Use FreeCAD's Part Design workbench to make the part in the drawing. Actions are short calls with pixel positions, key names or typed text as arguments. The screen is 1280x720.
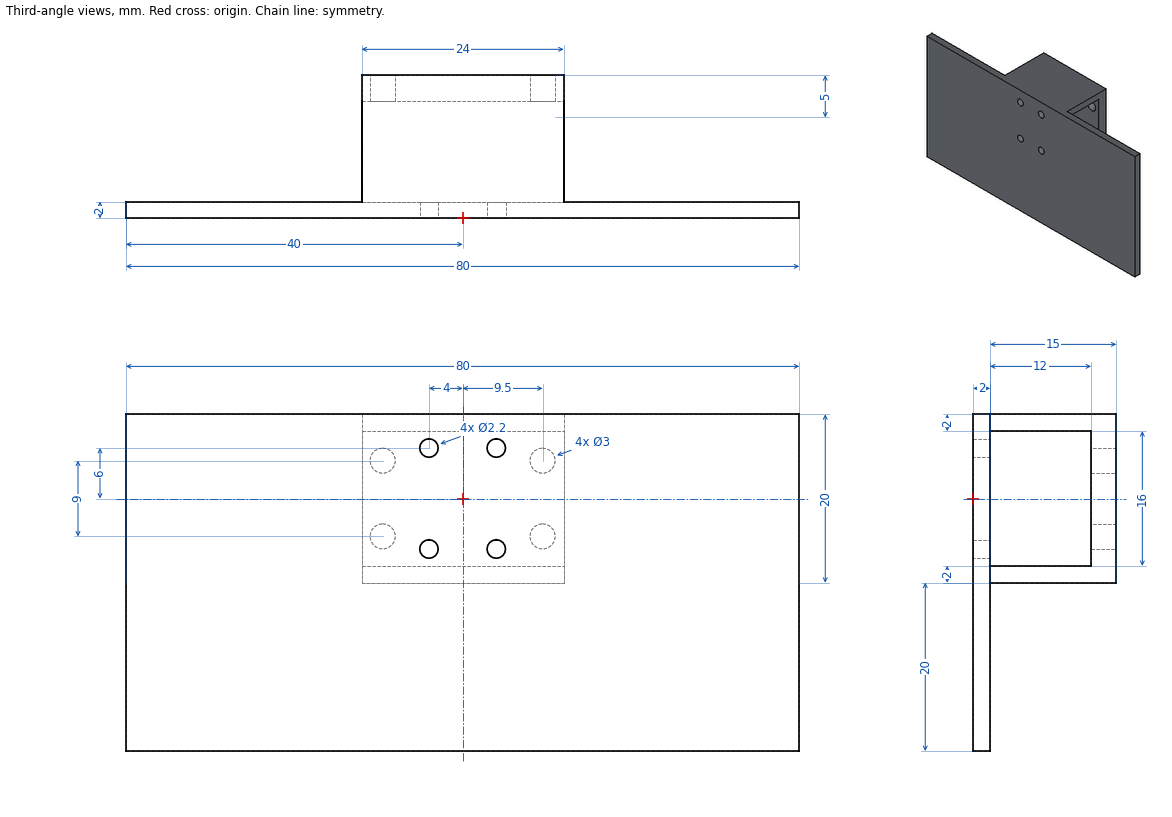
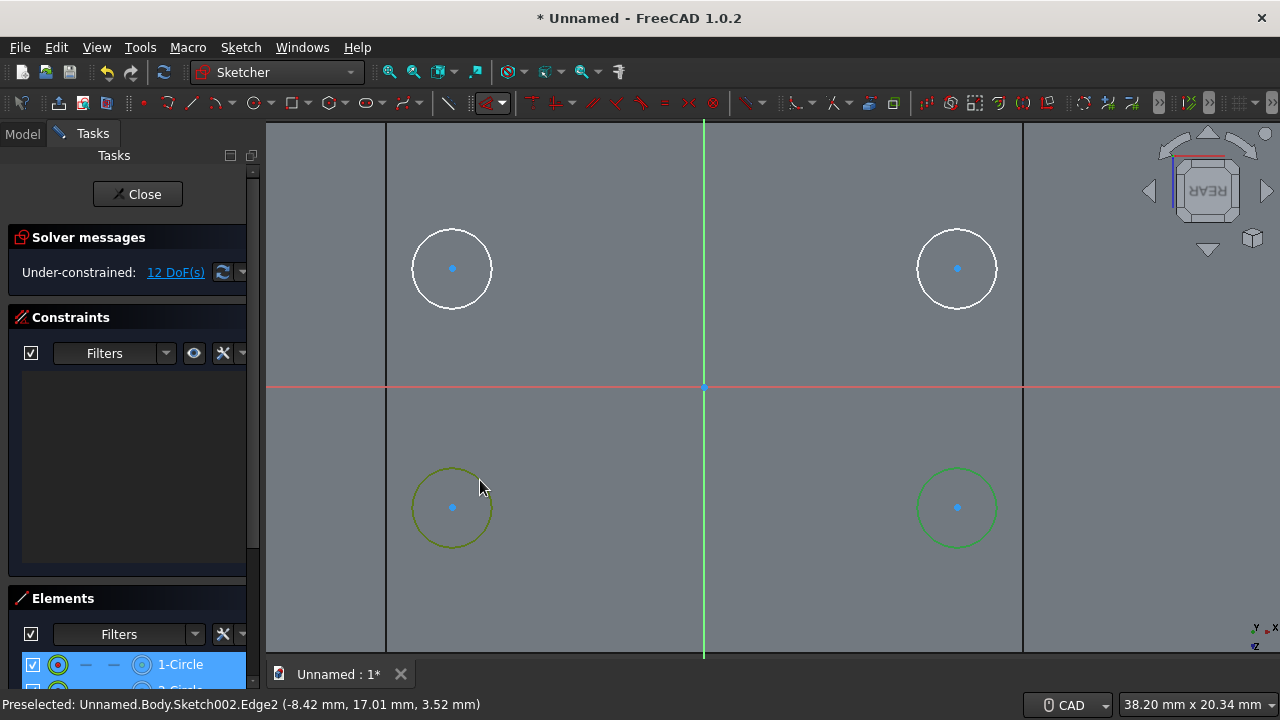
click(480, 241)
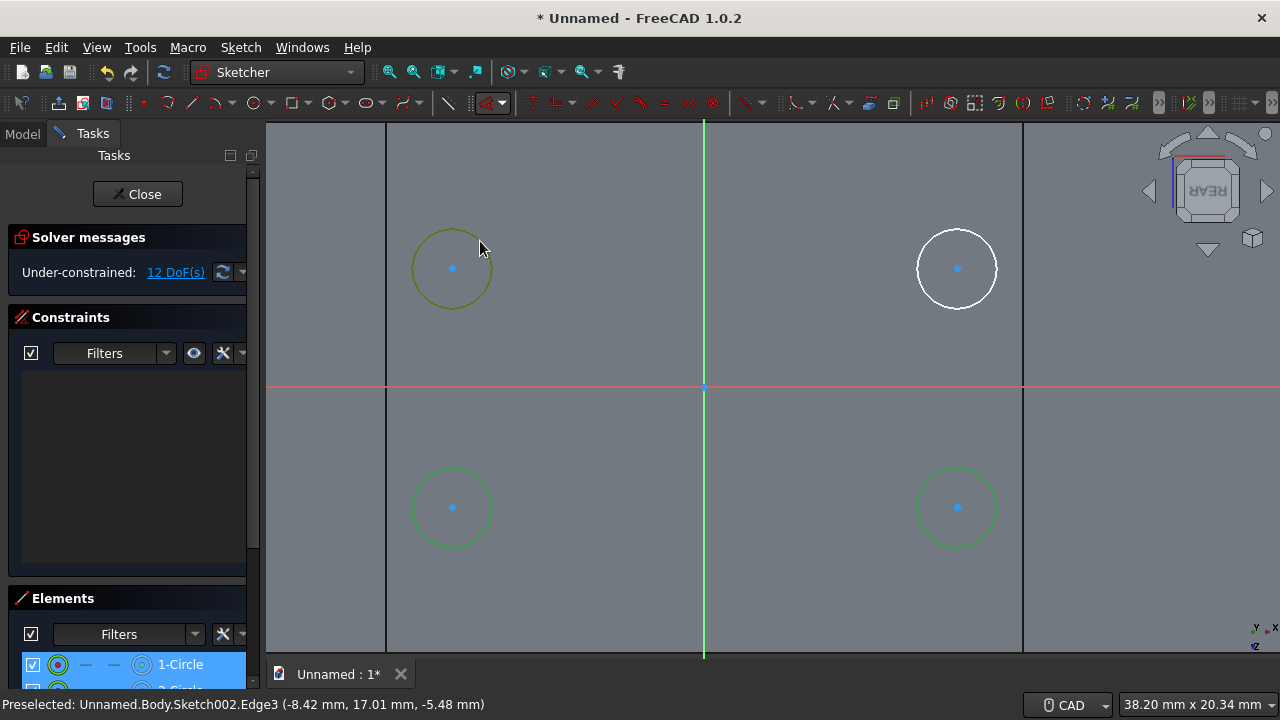
click(985, 241)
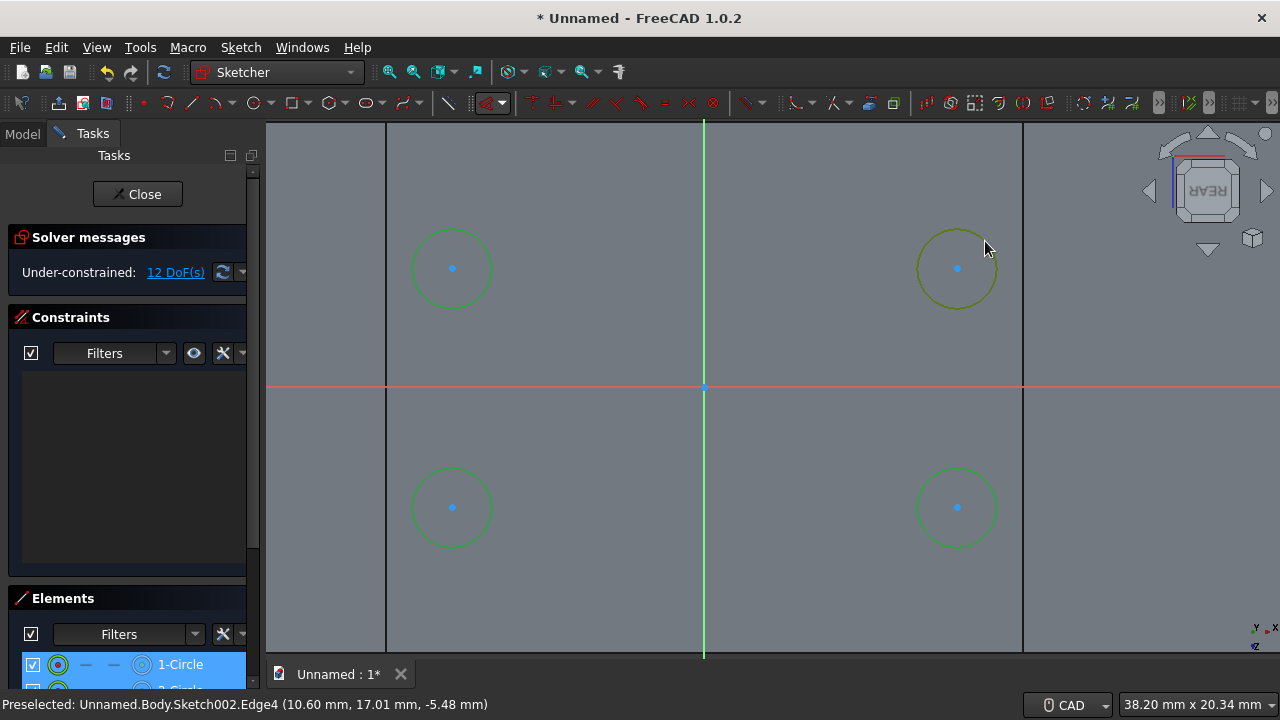
click(666, 104)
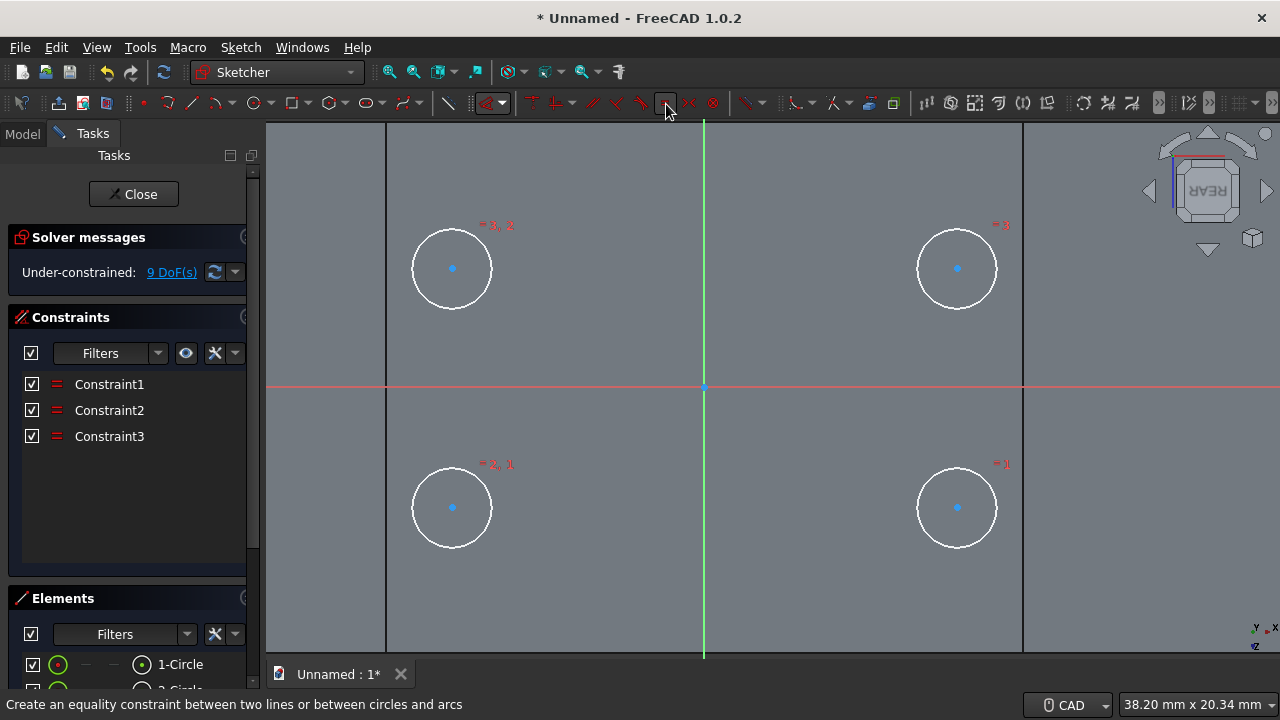
click(957, 508)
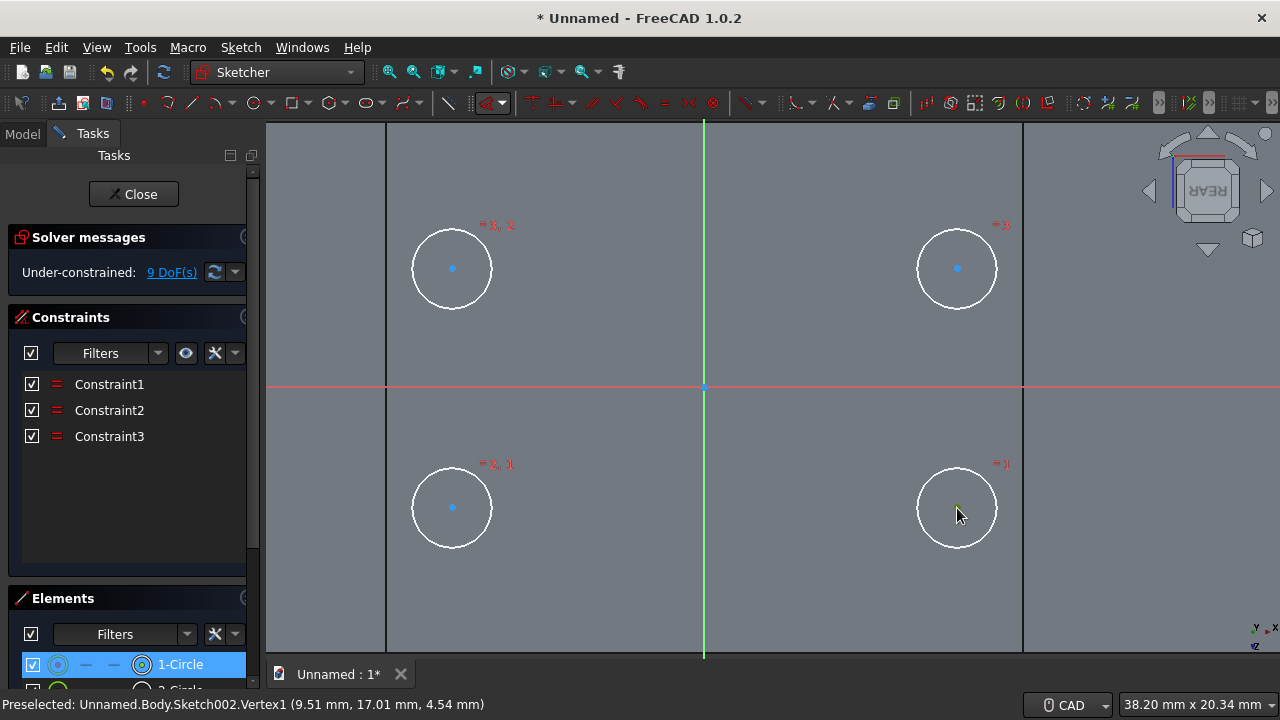
click(452, 508)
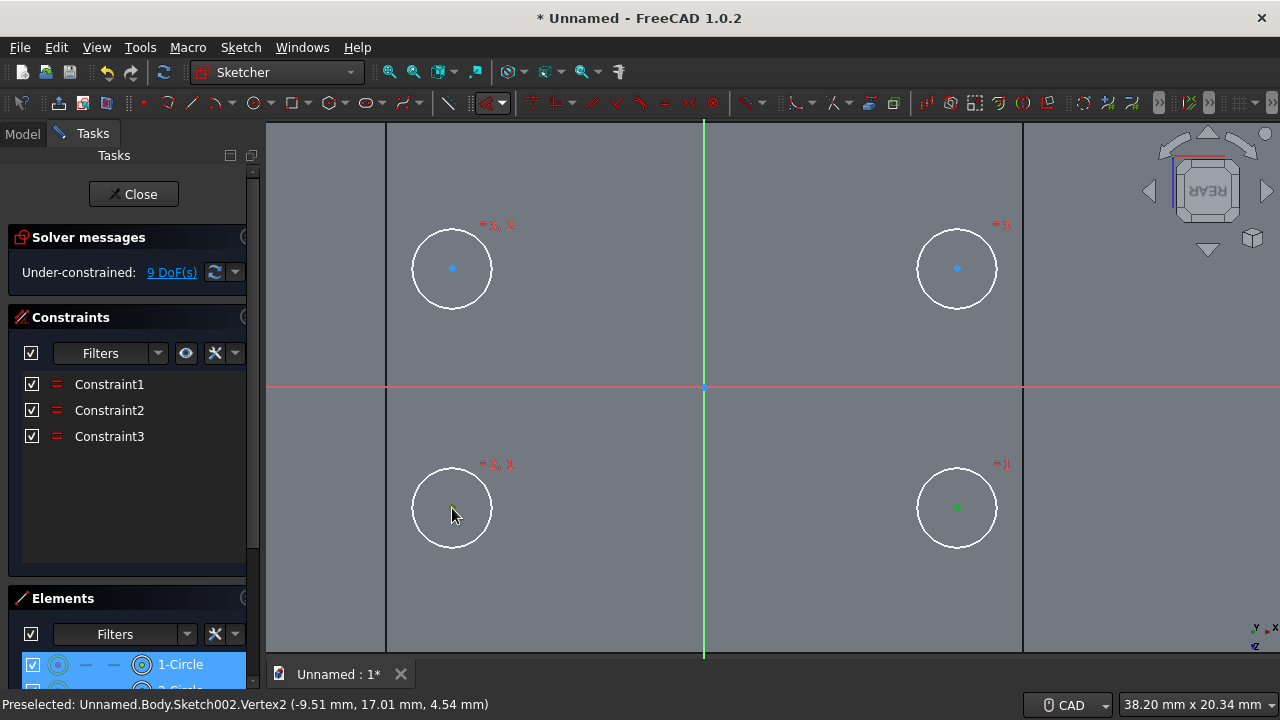
click(704, 596)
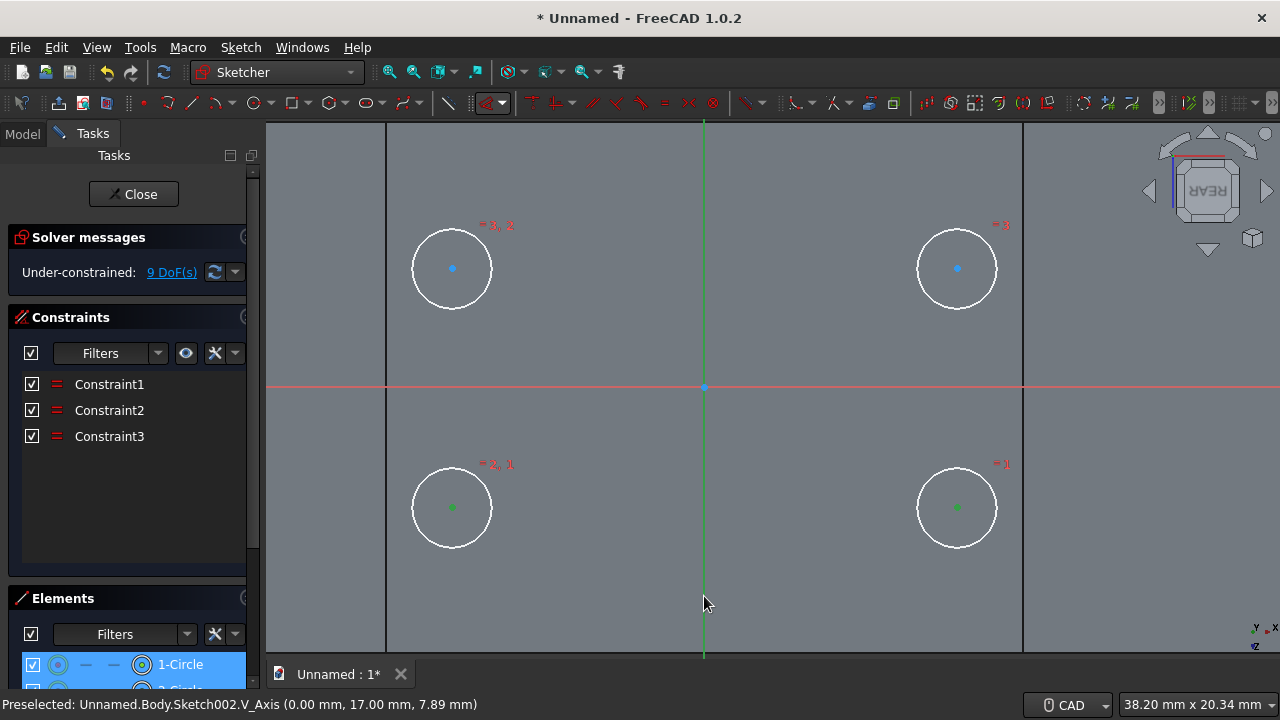
click(690, 104)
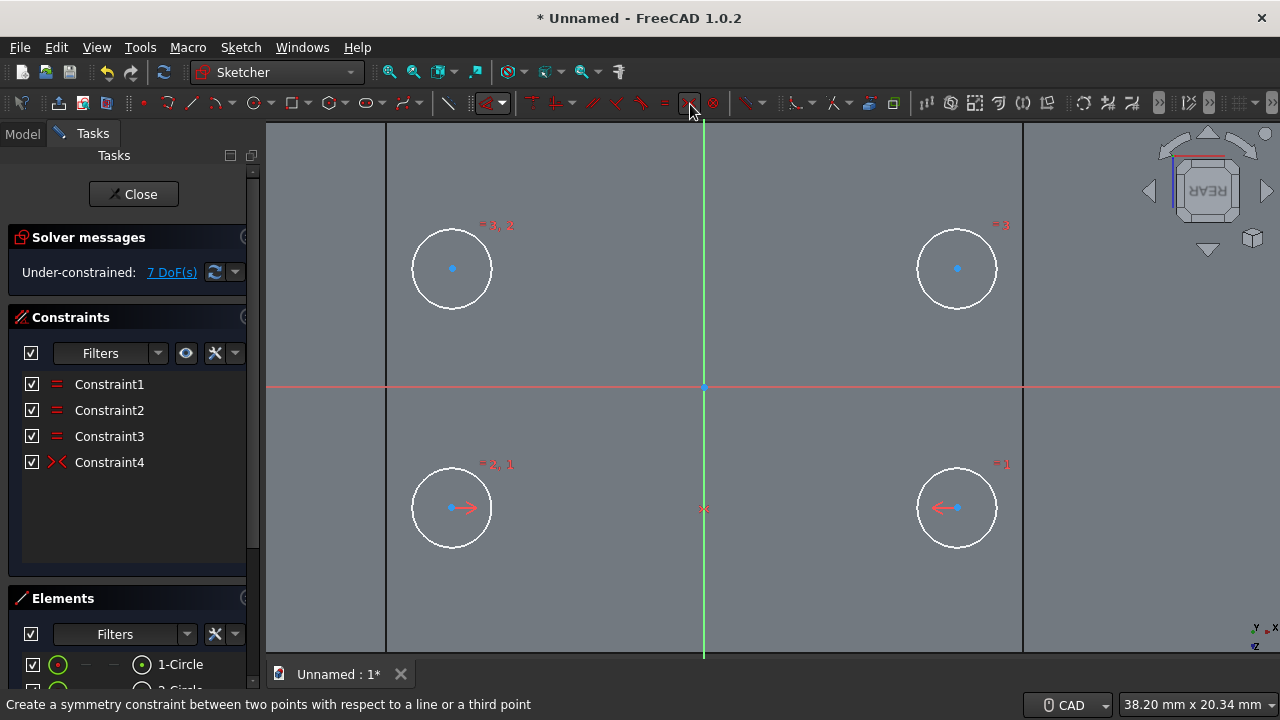
click(452, 508)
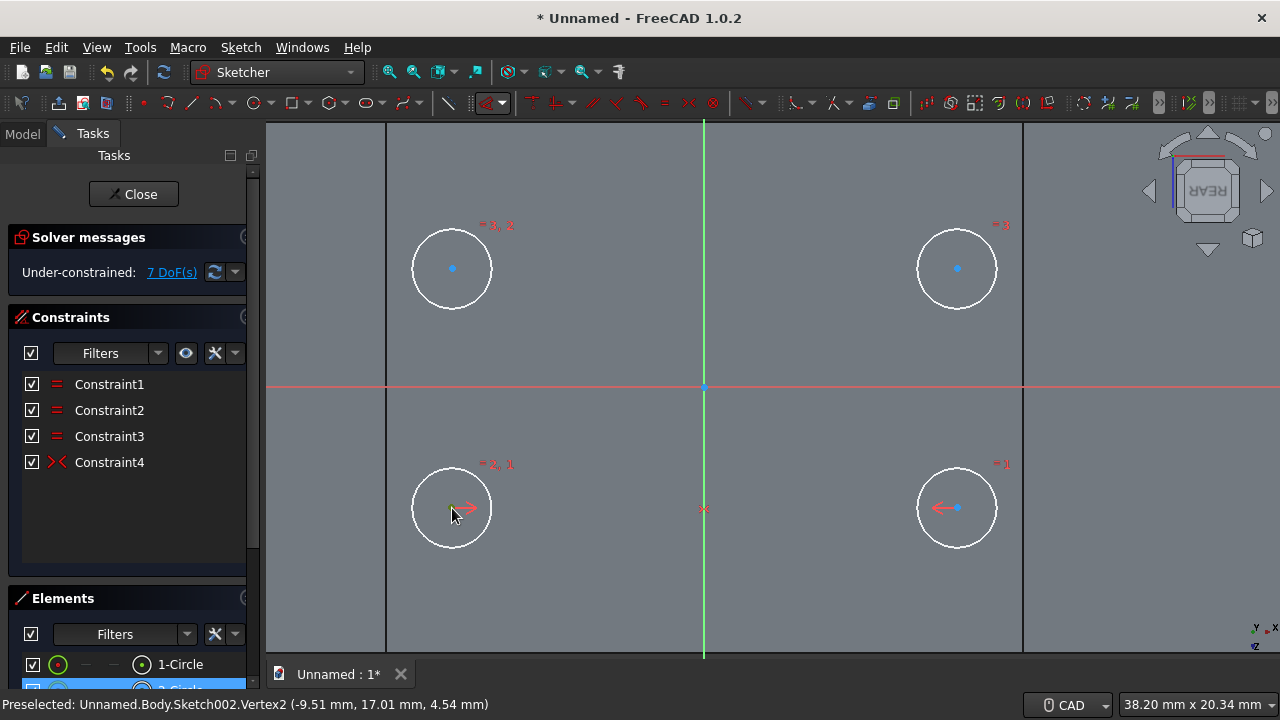
click(452, 269)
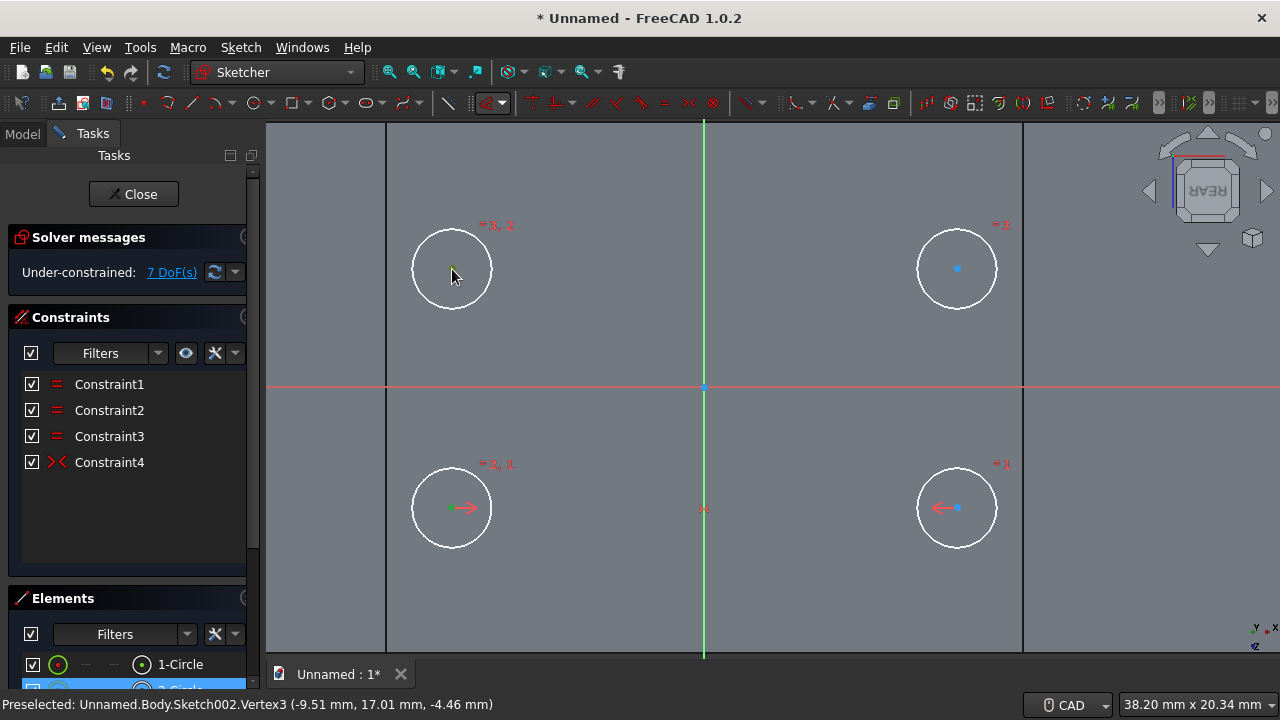
click(353, 387)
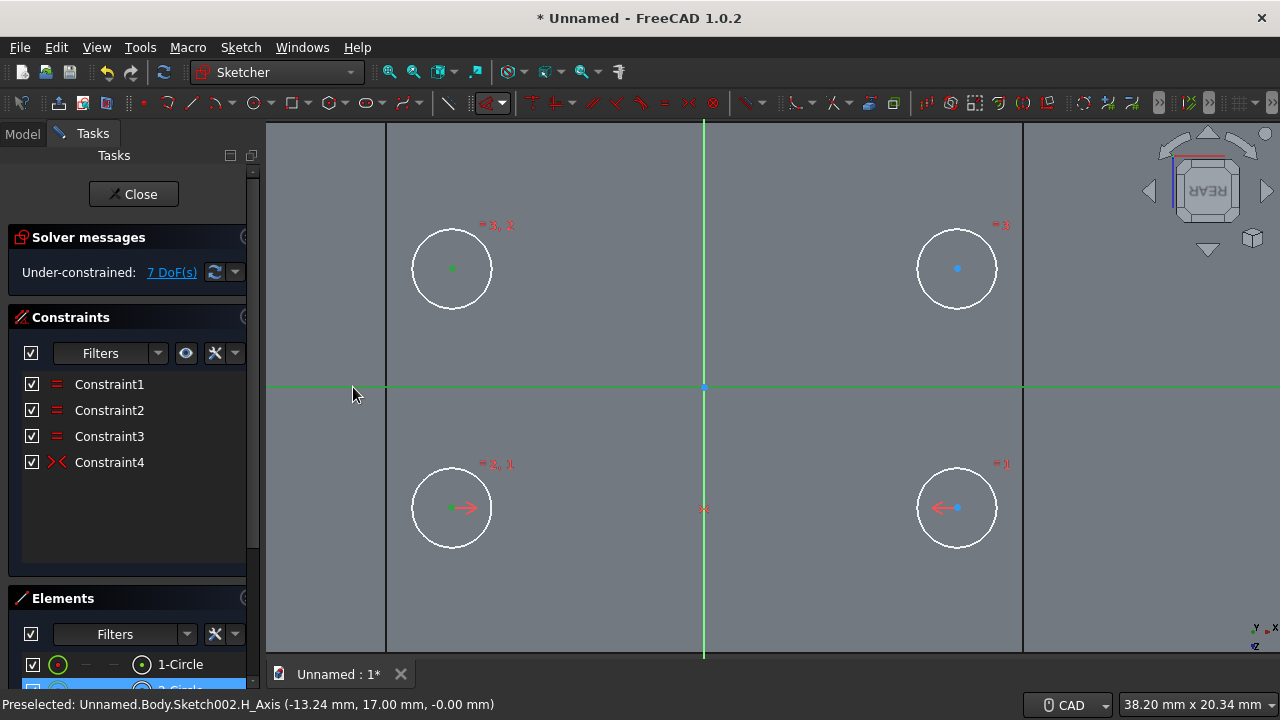
click(690, 104)